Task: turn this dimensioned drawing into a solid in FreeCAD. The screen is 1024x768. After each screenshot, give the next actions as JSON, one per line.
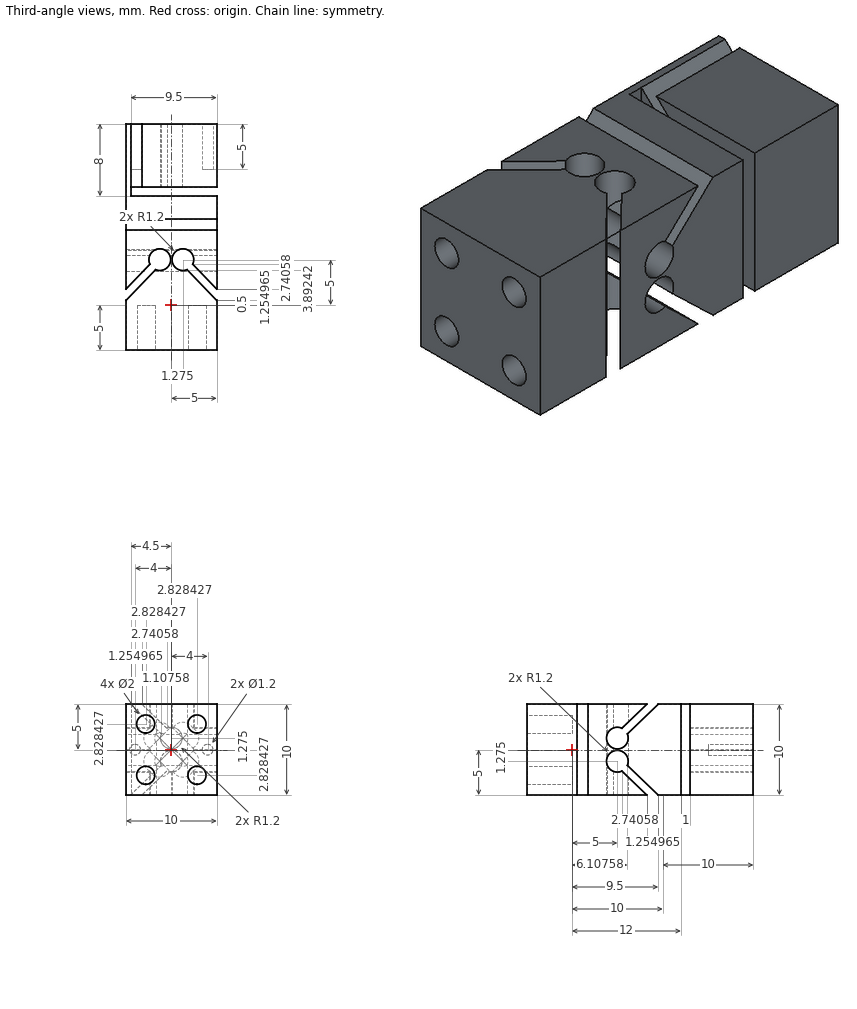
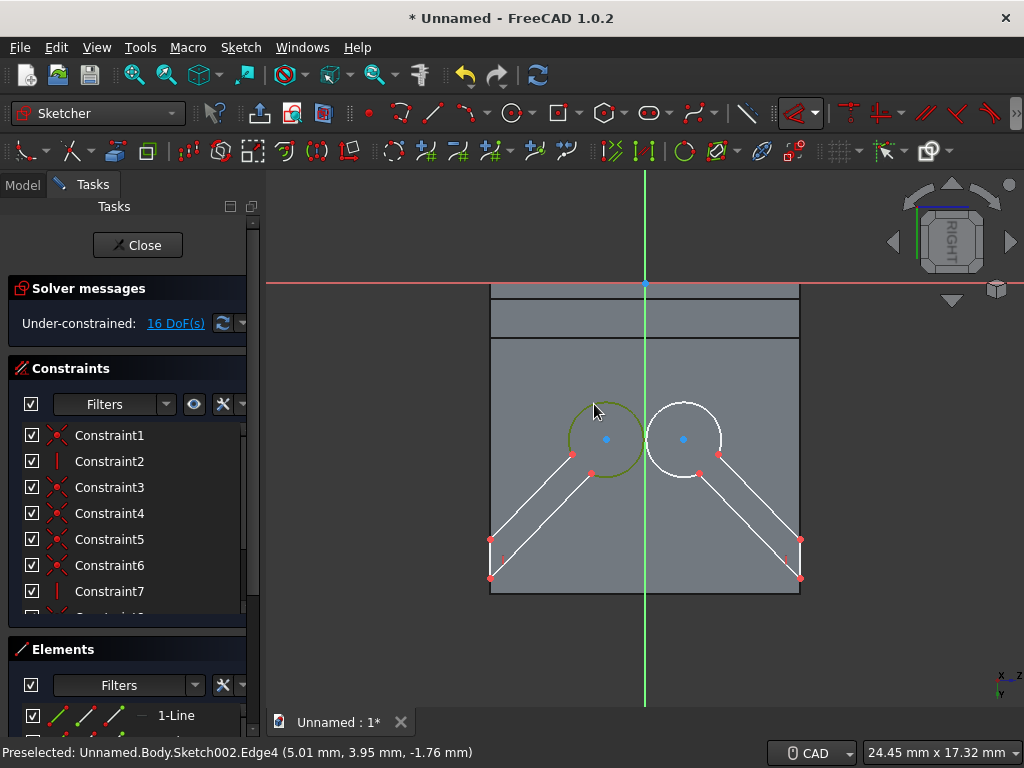
{"action": "left_click", "coordinate": [696, 404]}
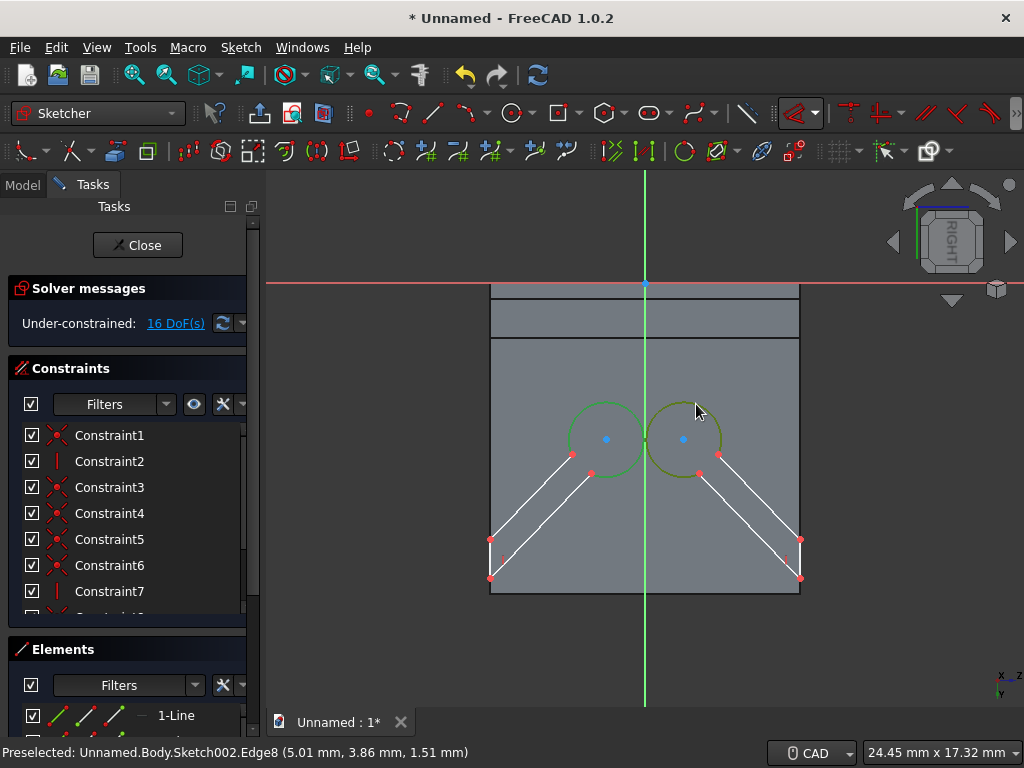
{"action": "key", "text": "e"}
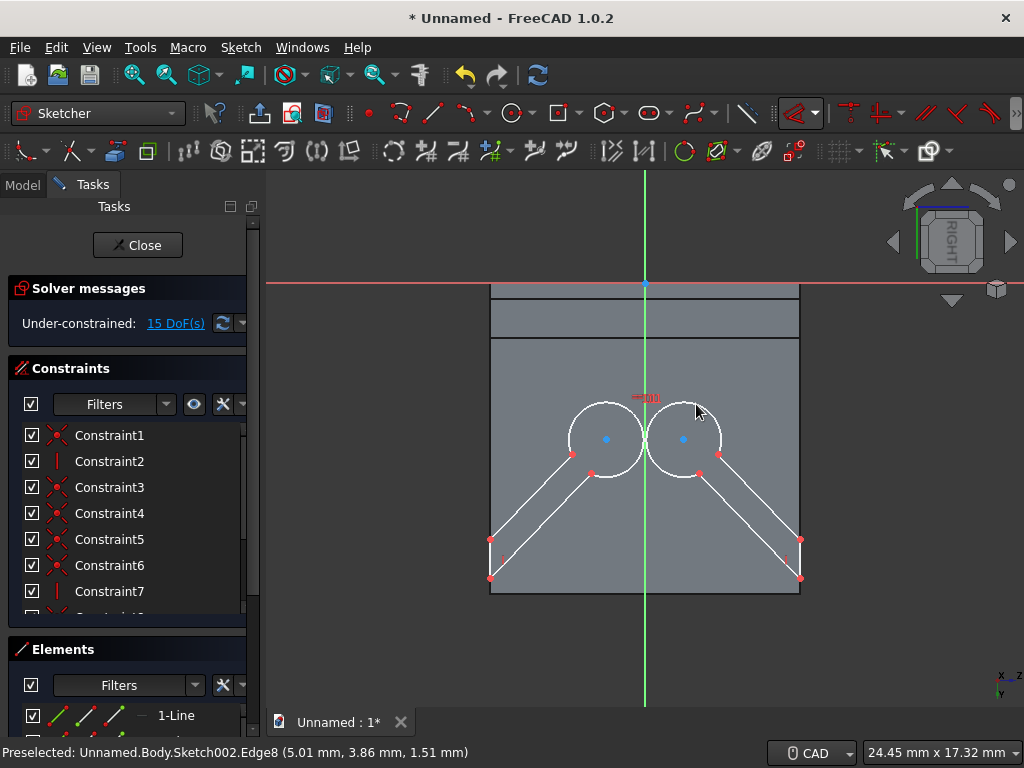
{"action": "left_click", "coordinate": [606, 440]}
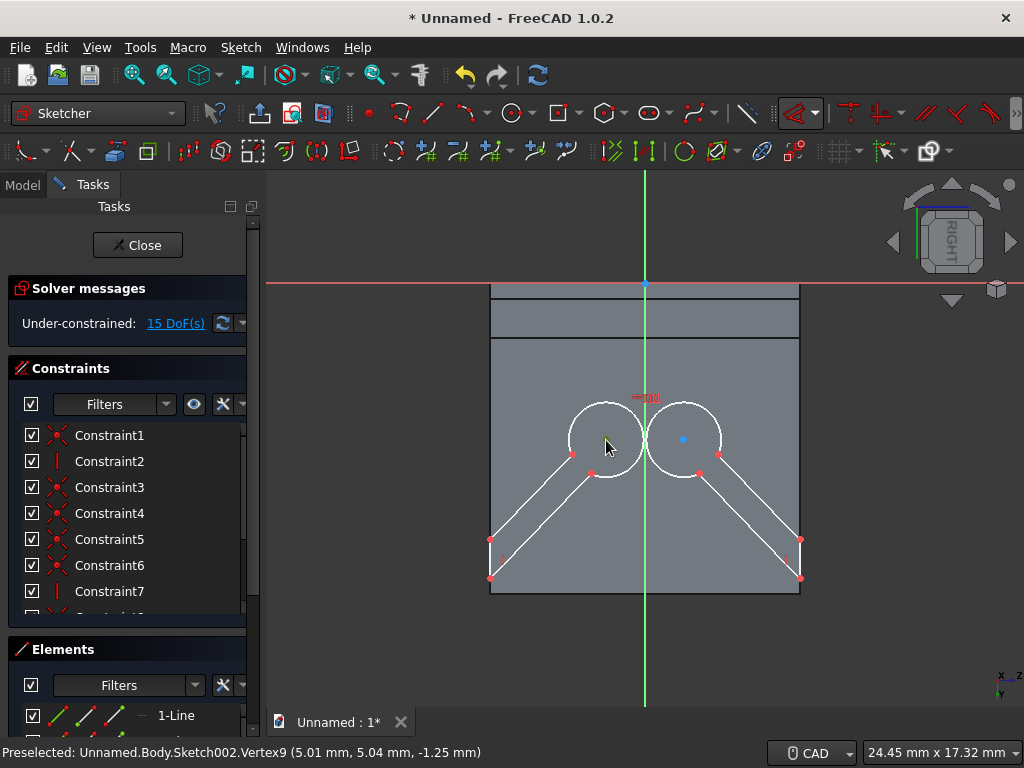
{"action": "left_click", "coordinate": [684, 440]}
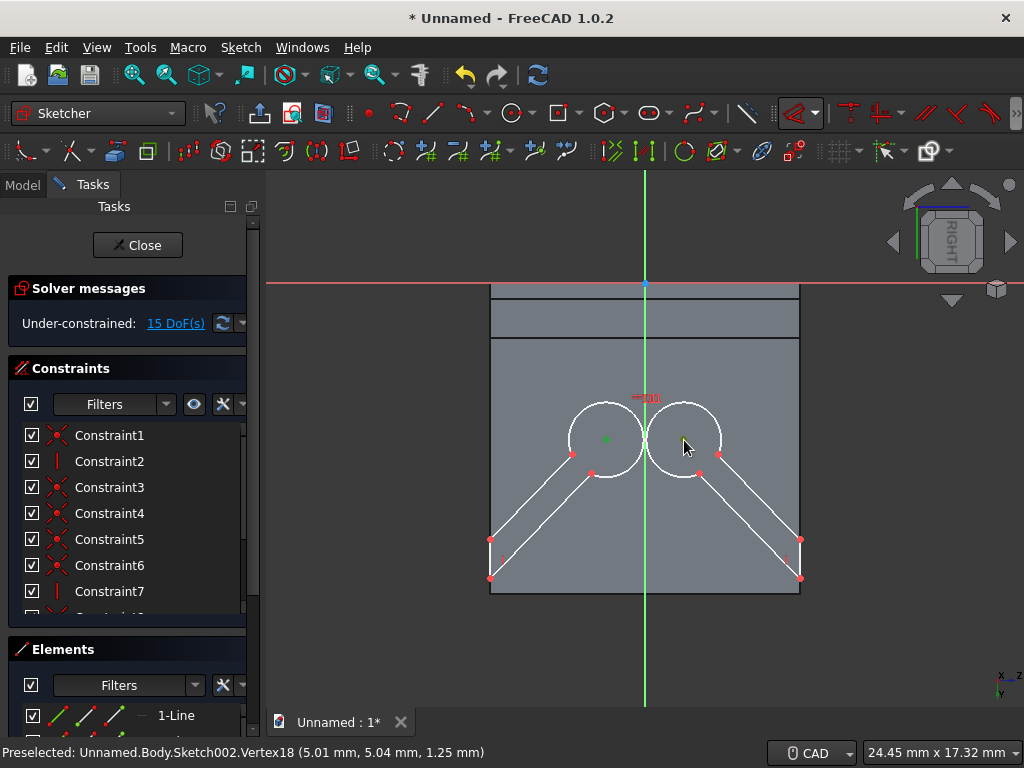
{"action": "left_click", "coordinate": [645, 645]}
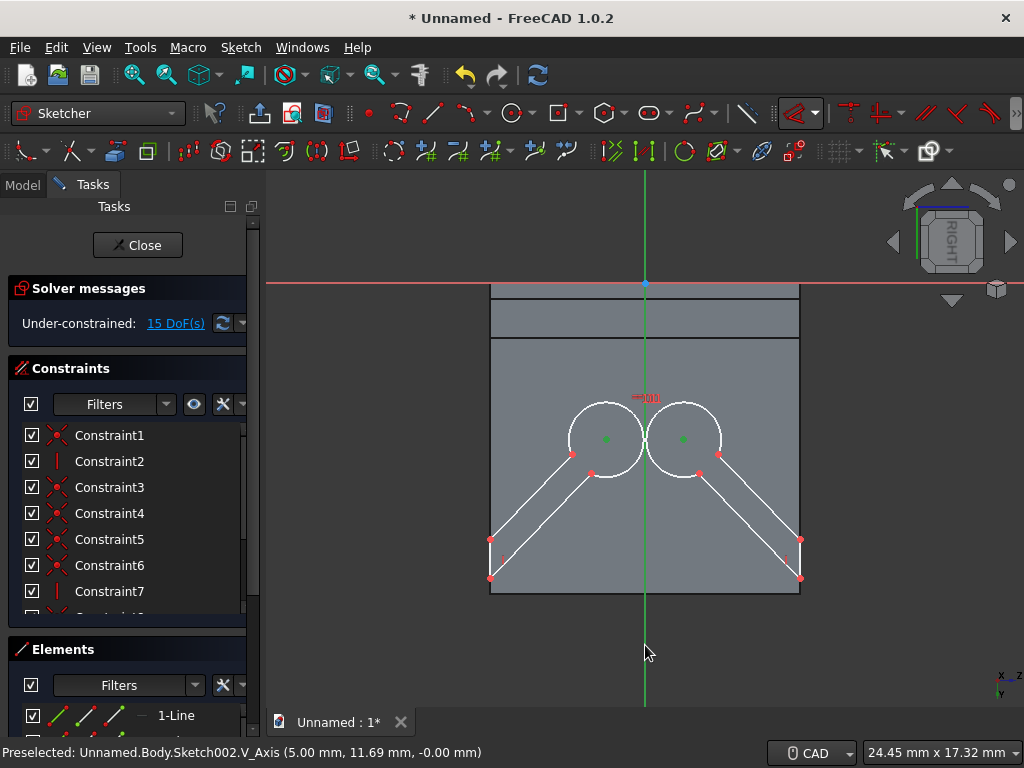
{"action": "key", "text": "s"}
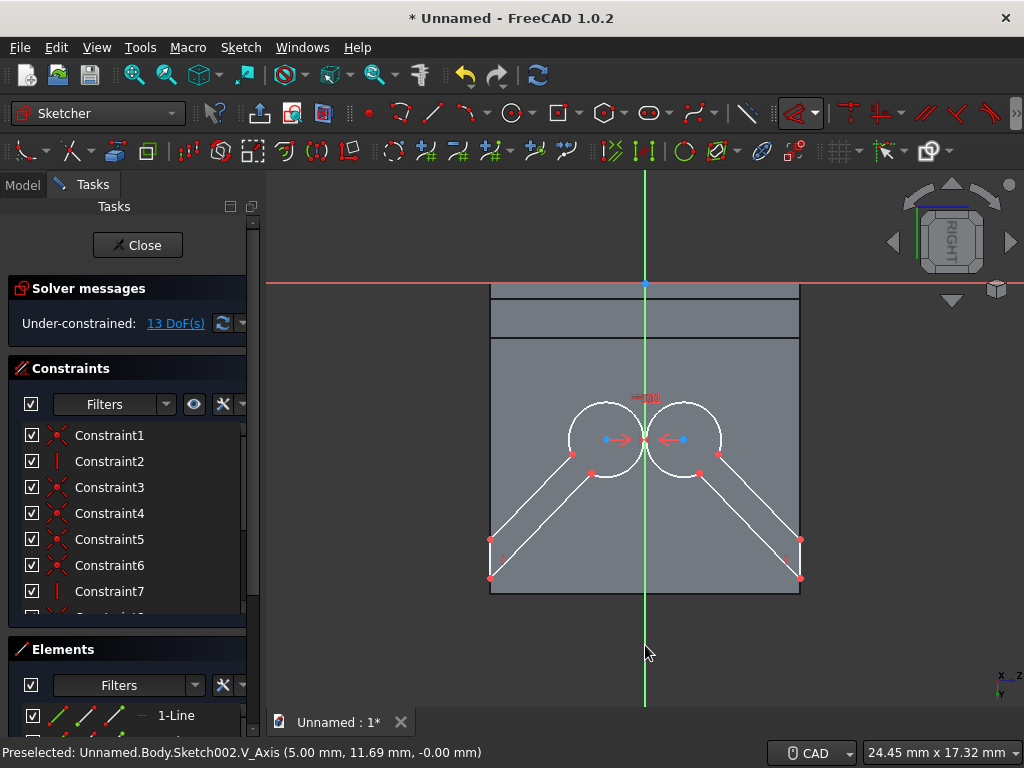
{"action": "left_click", "coordinate": [490, 579]}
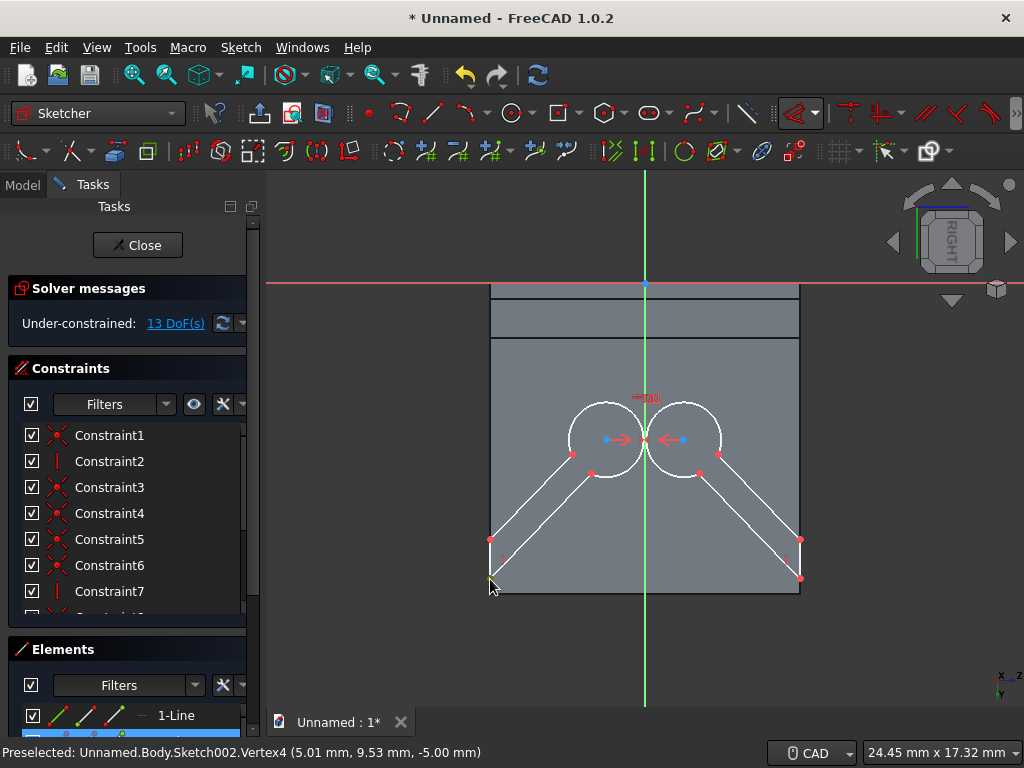
{"action": "left_click", "coordinate": [800, 579]}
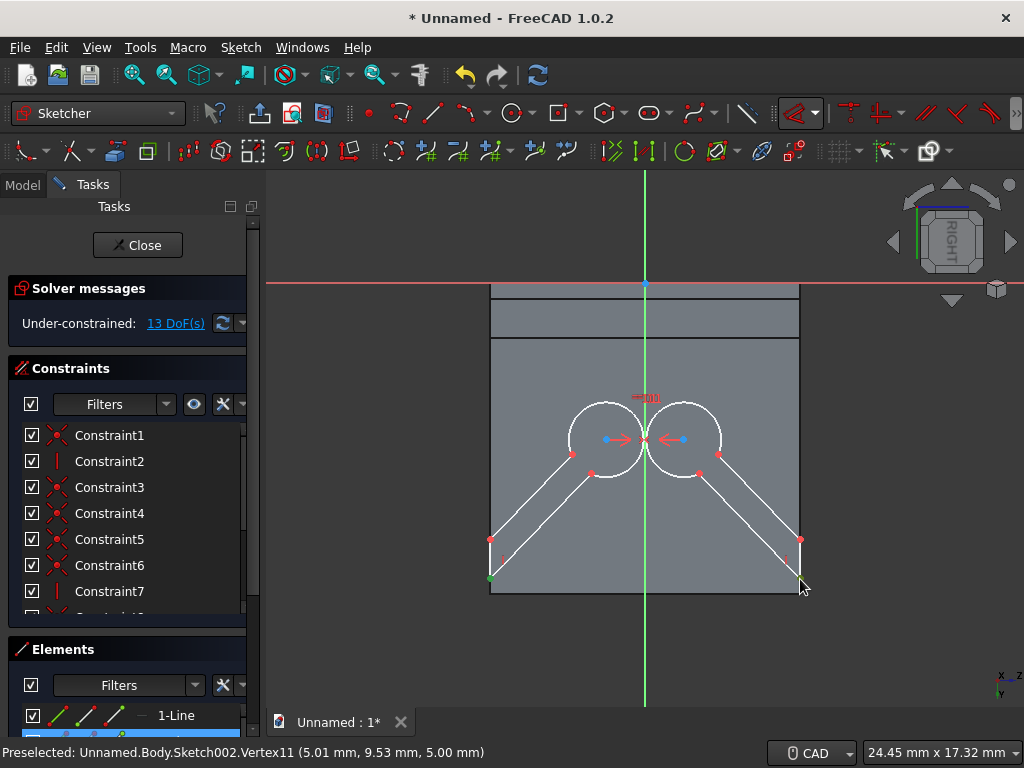
{"action": "left_click", "coordinate": [645, 645]}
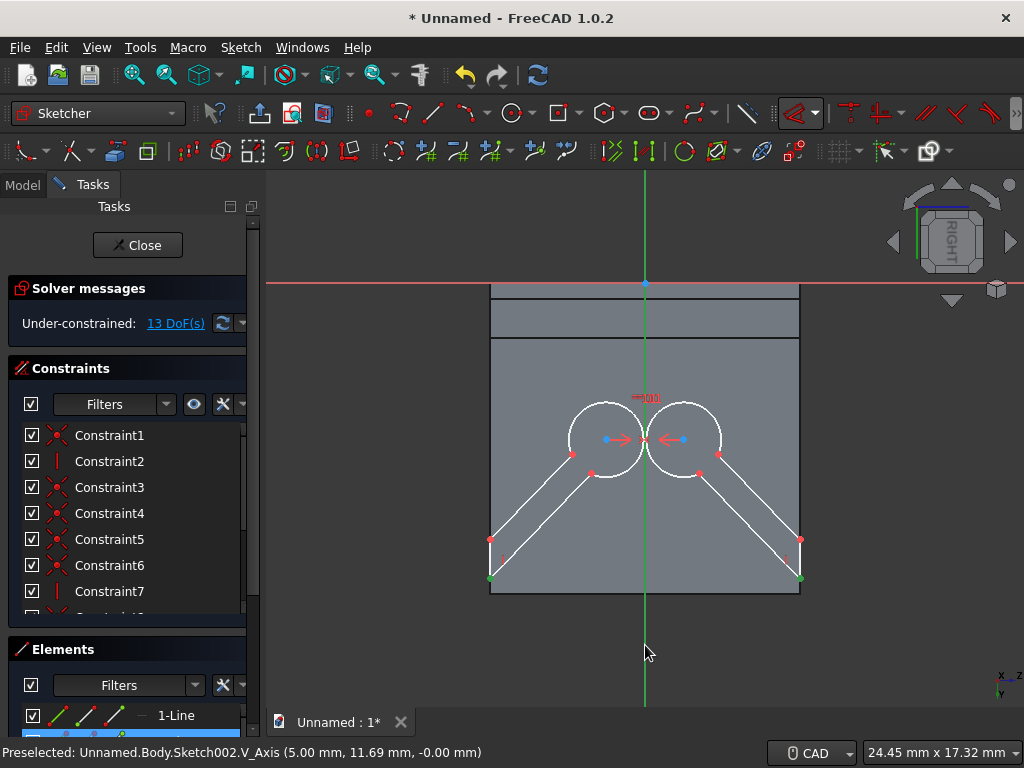
{"action": "key", "text": "s"}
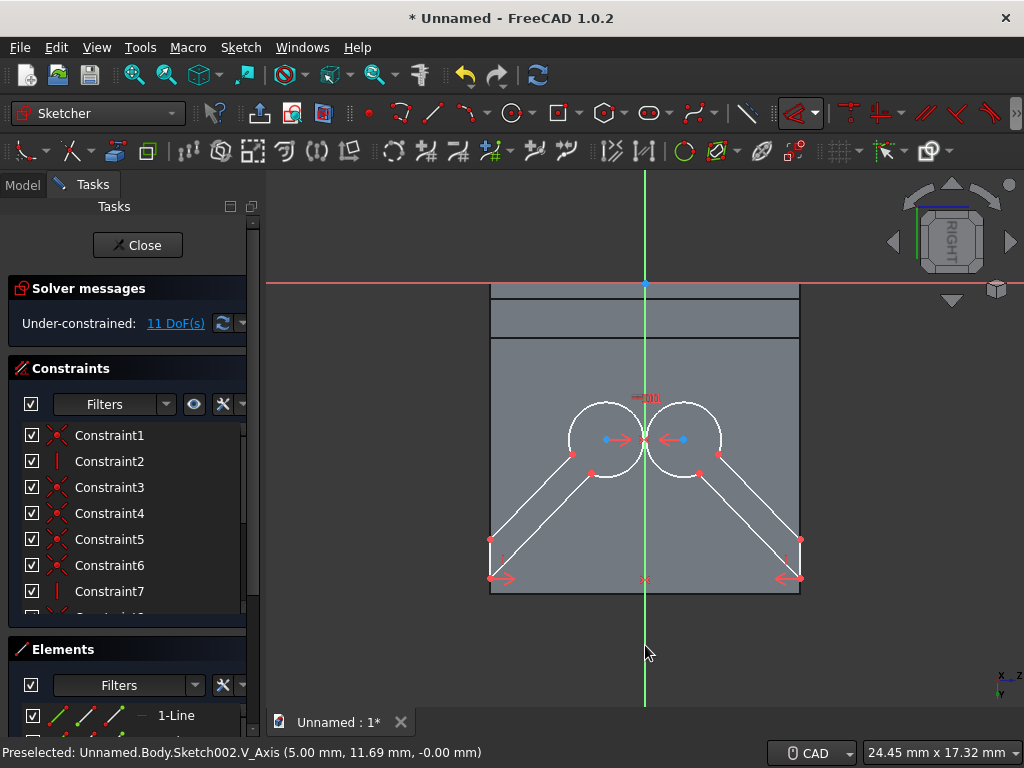
{"action": "left_click", "coordinate": [594, 404]}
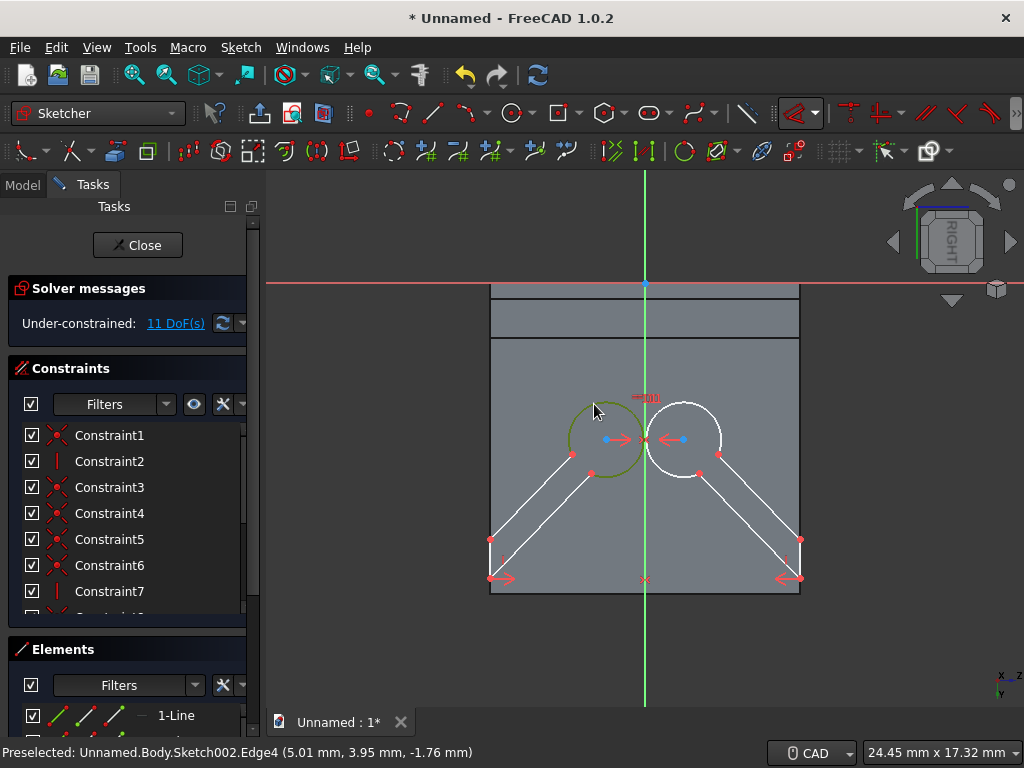
{"action": "key", "text": "k r"}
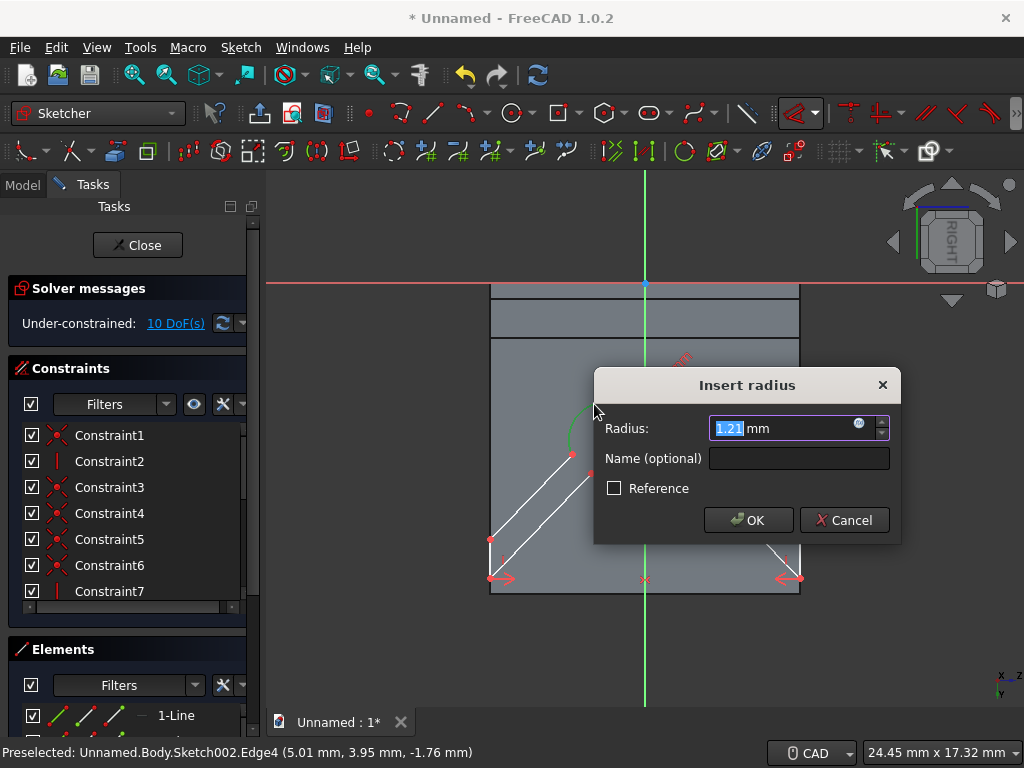
{"action": "type", "text": "1.2"}
{"action": "key", "text": "Return"}